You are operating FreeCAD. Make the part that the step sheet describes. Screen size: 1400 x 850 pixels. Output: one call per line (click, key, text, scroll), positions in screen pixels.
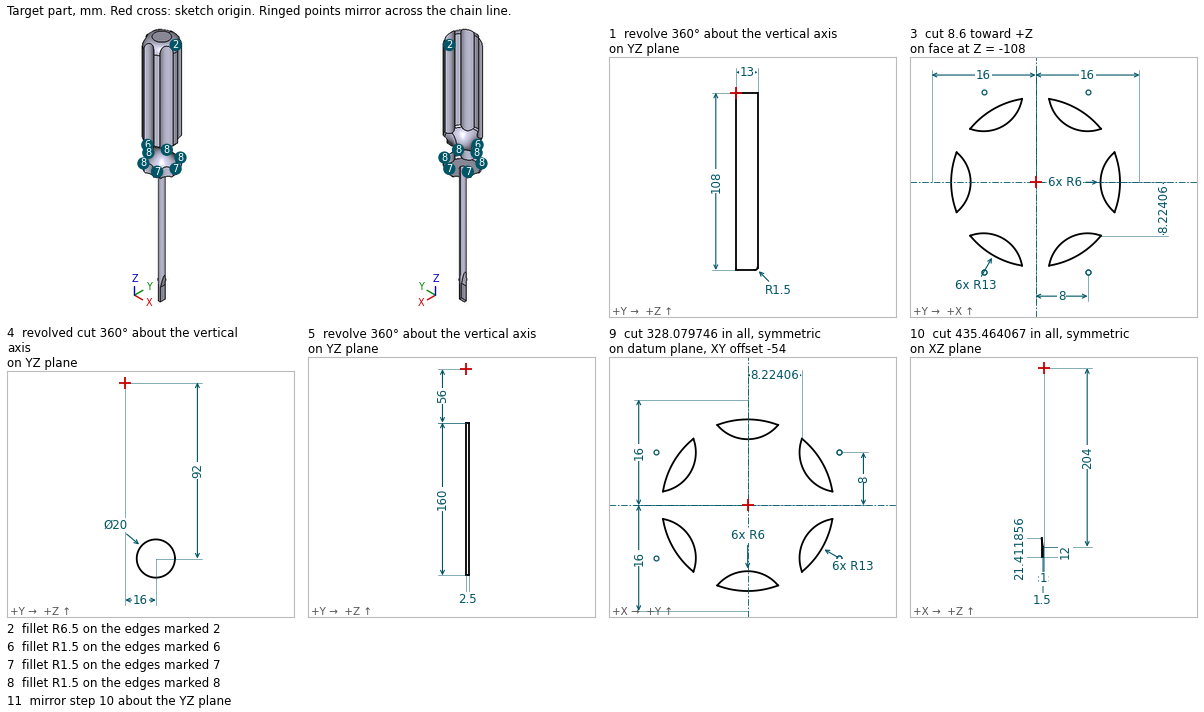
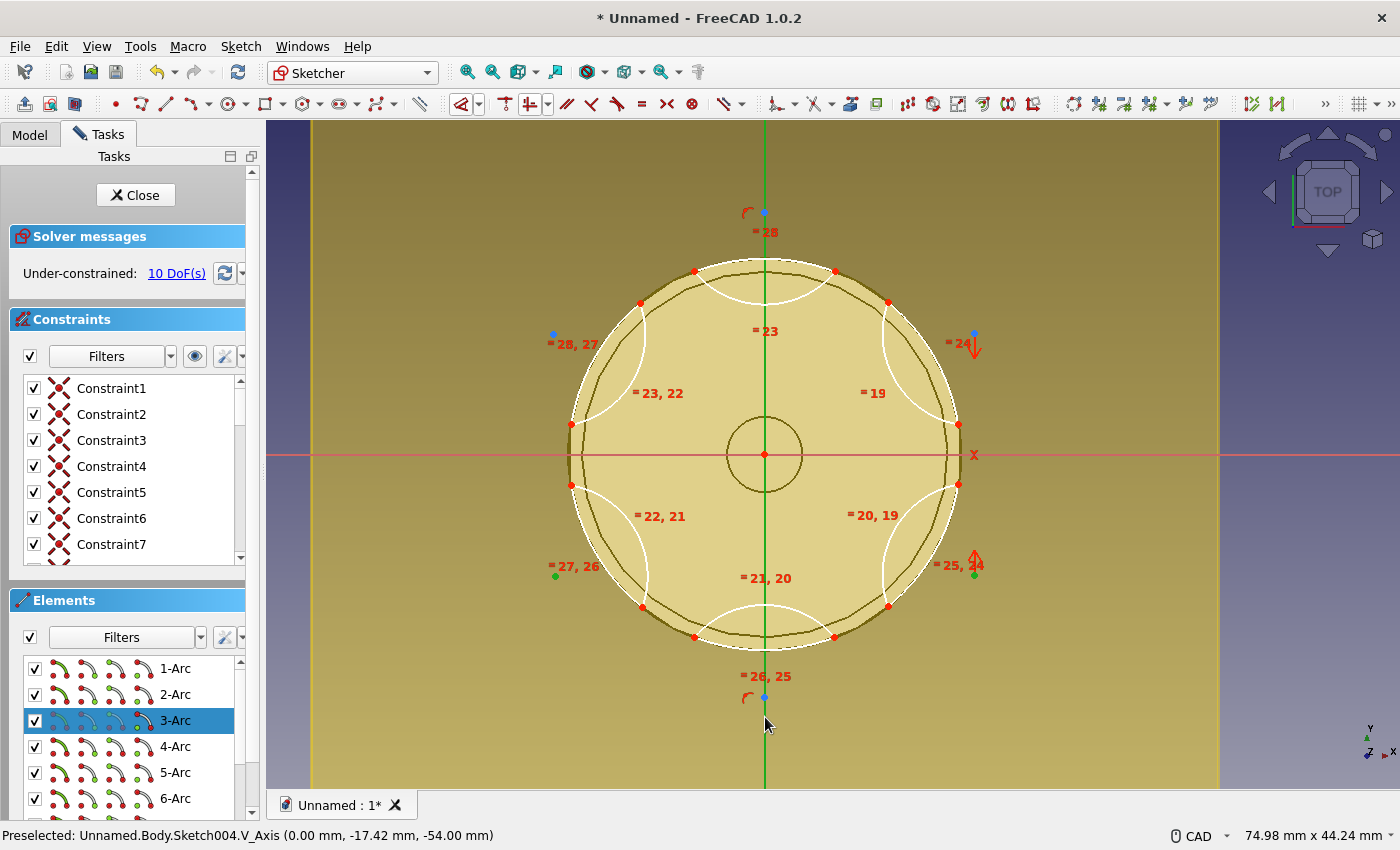
key(s)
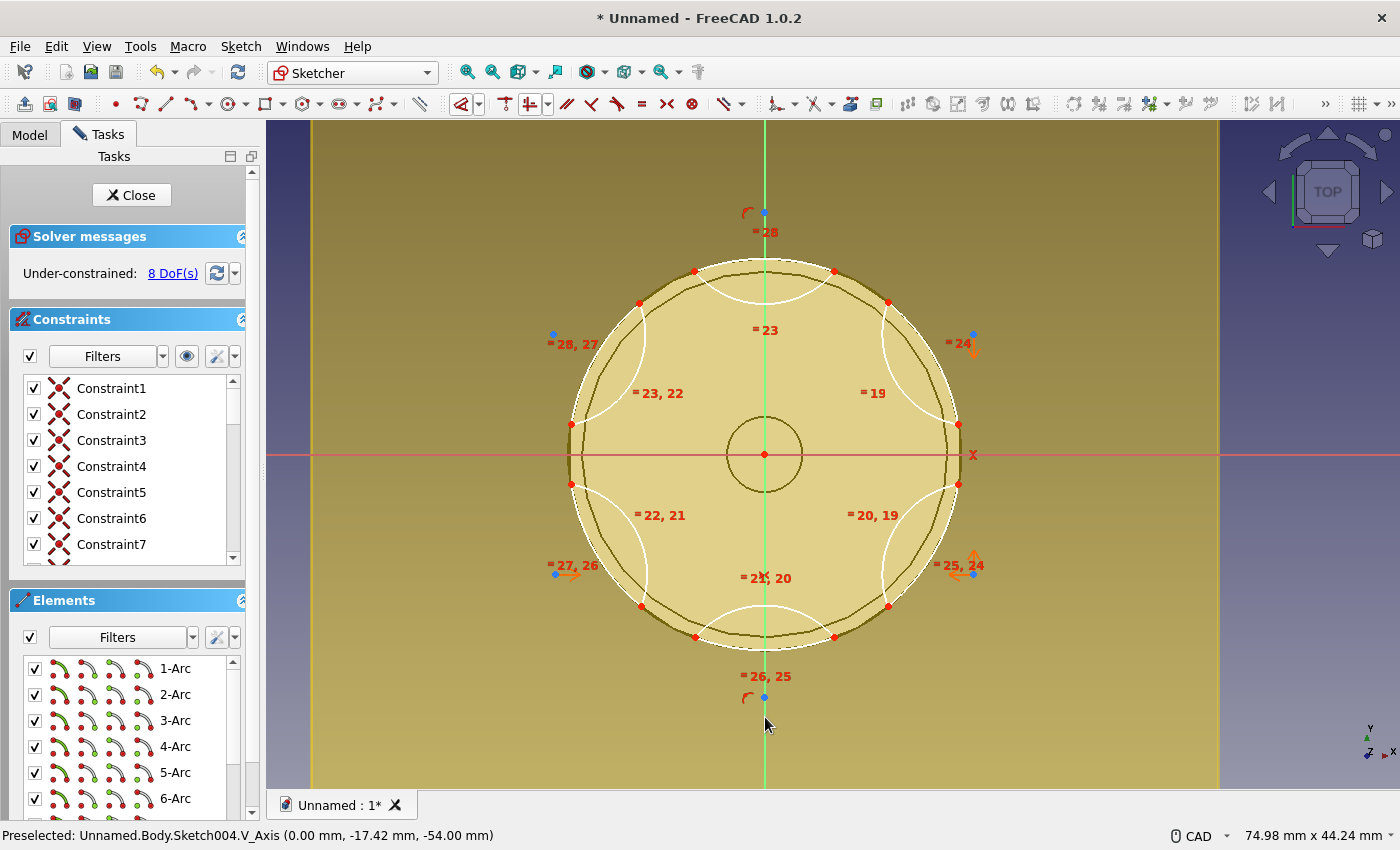
click(974, 334)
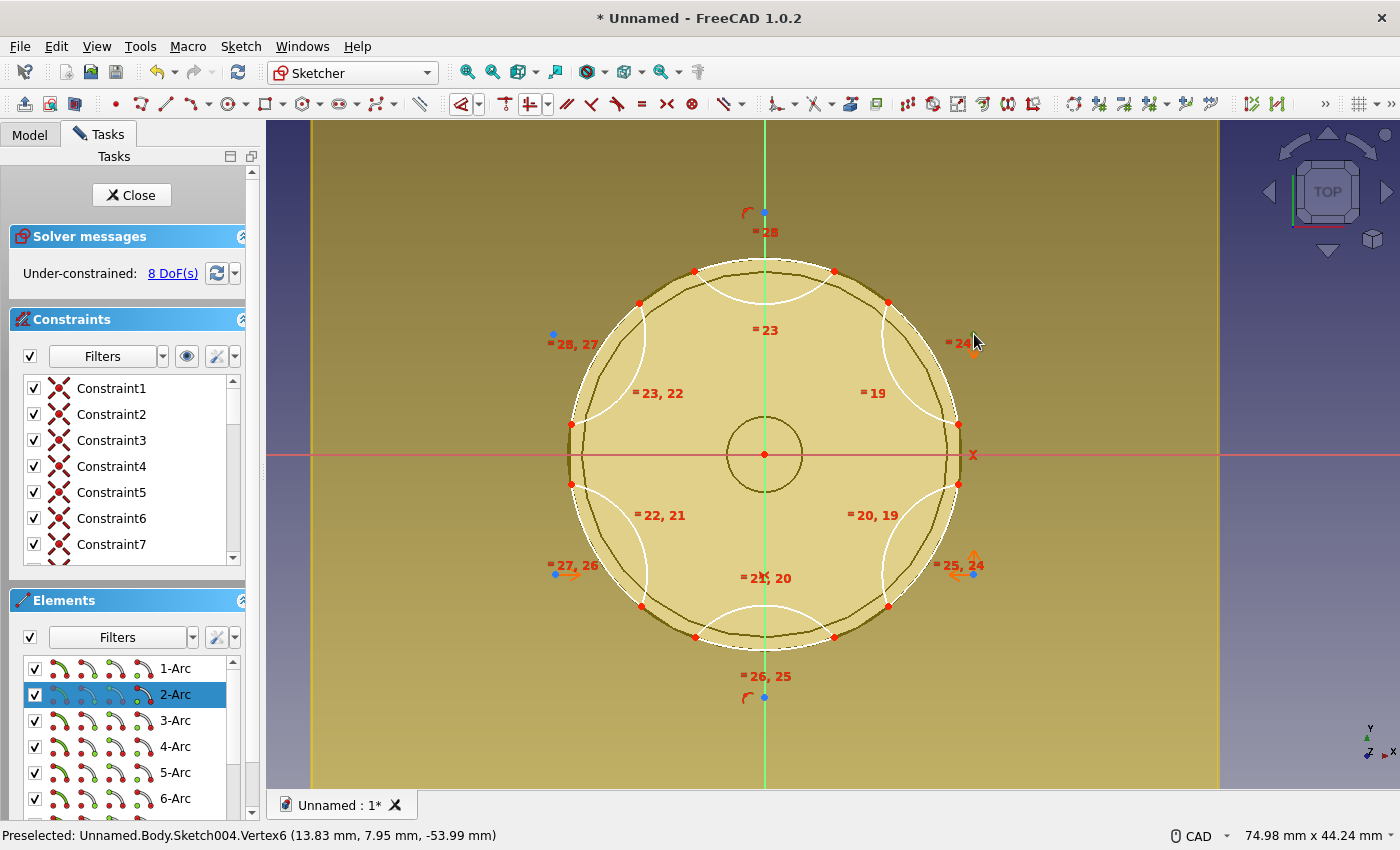
click(554, 335)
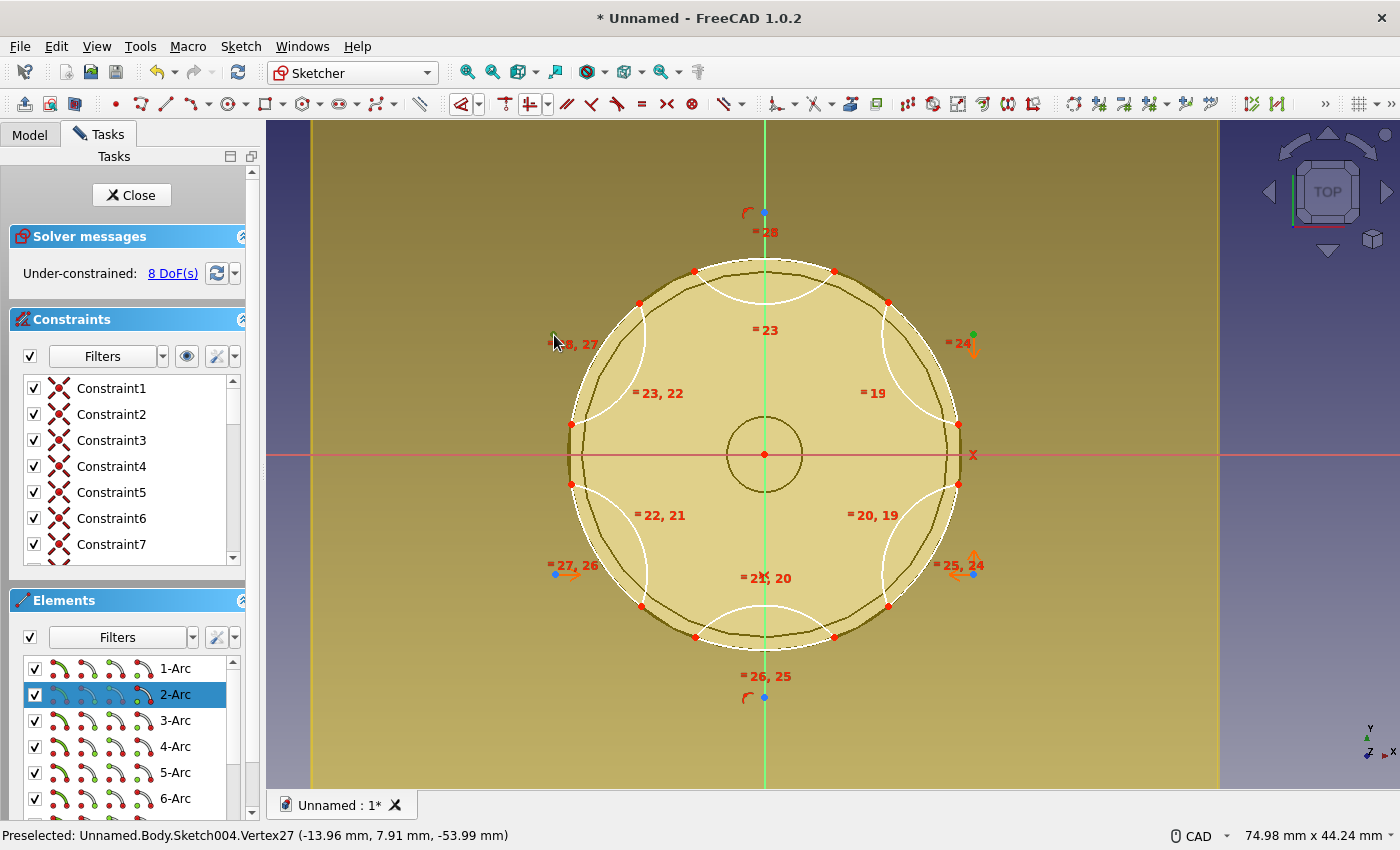
click(765, 717)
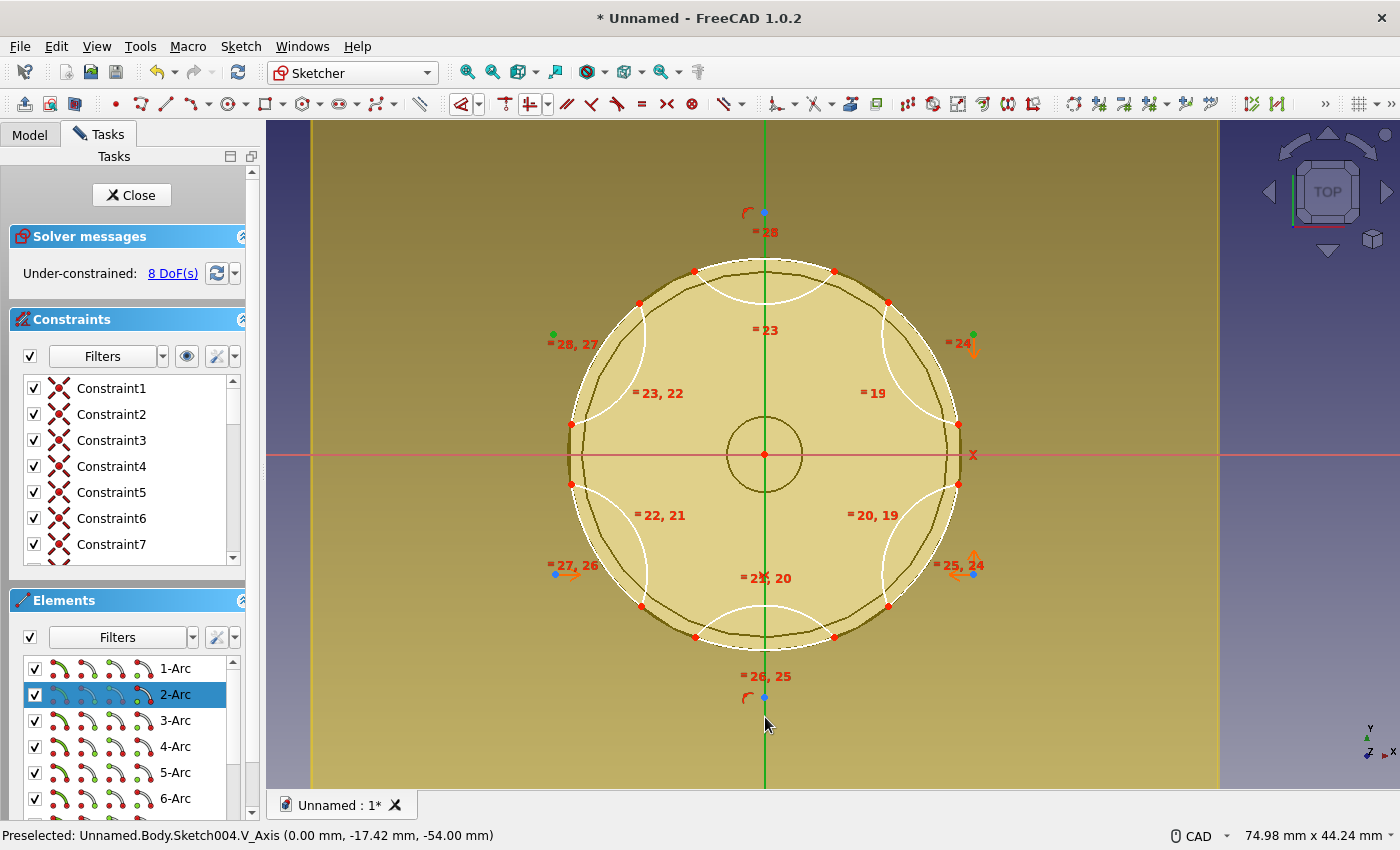
click(667, 104)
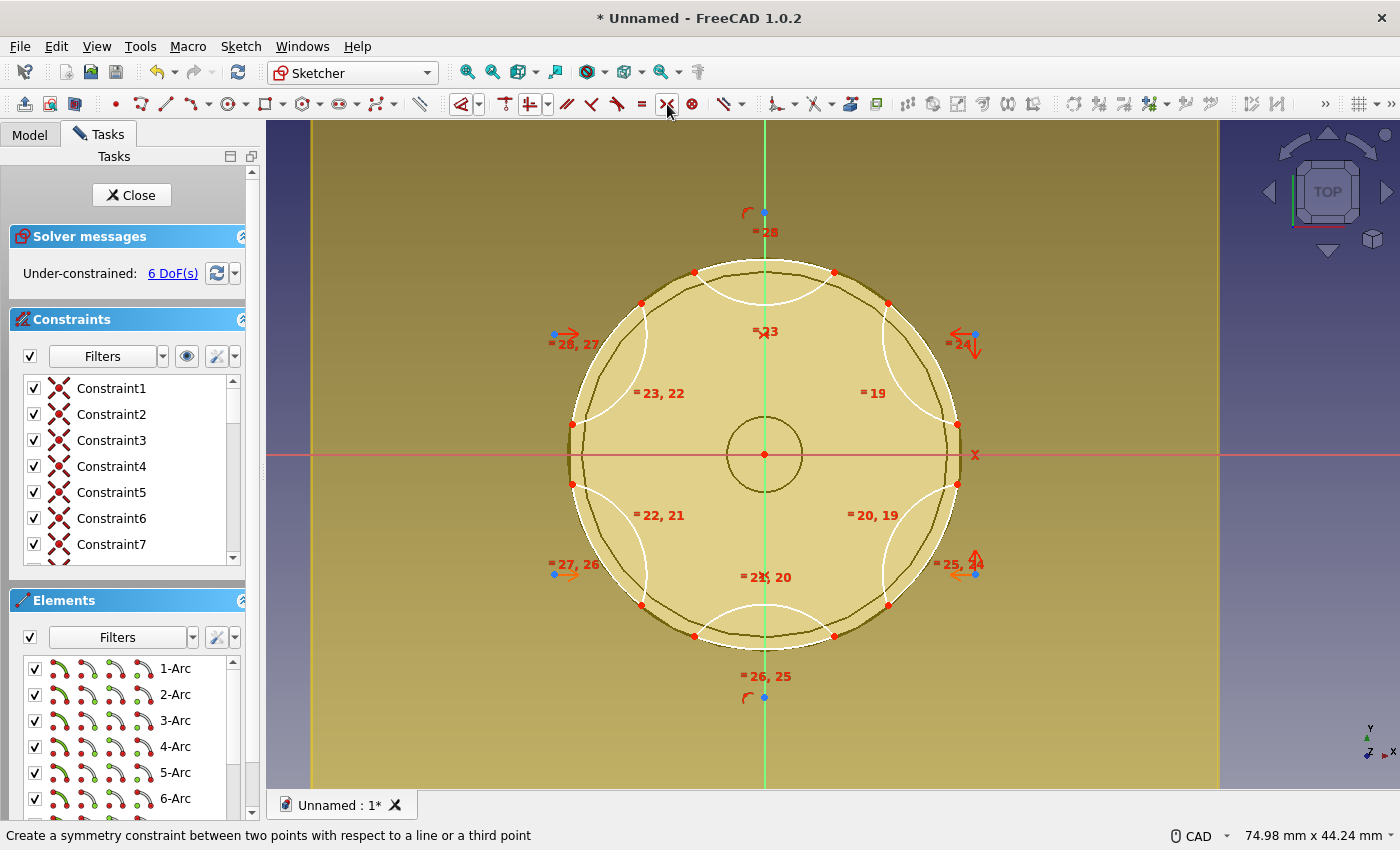
key(d)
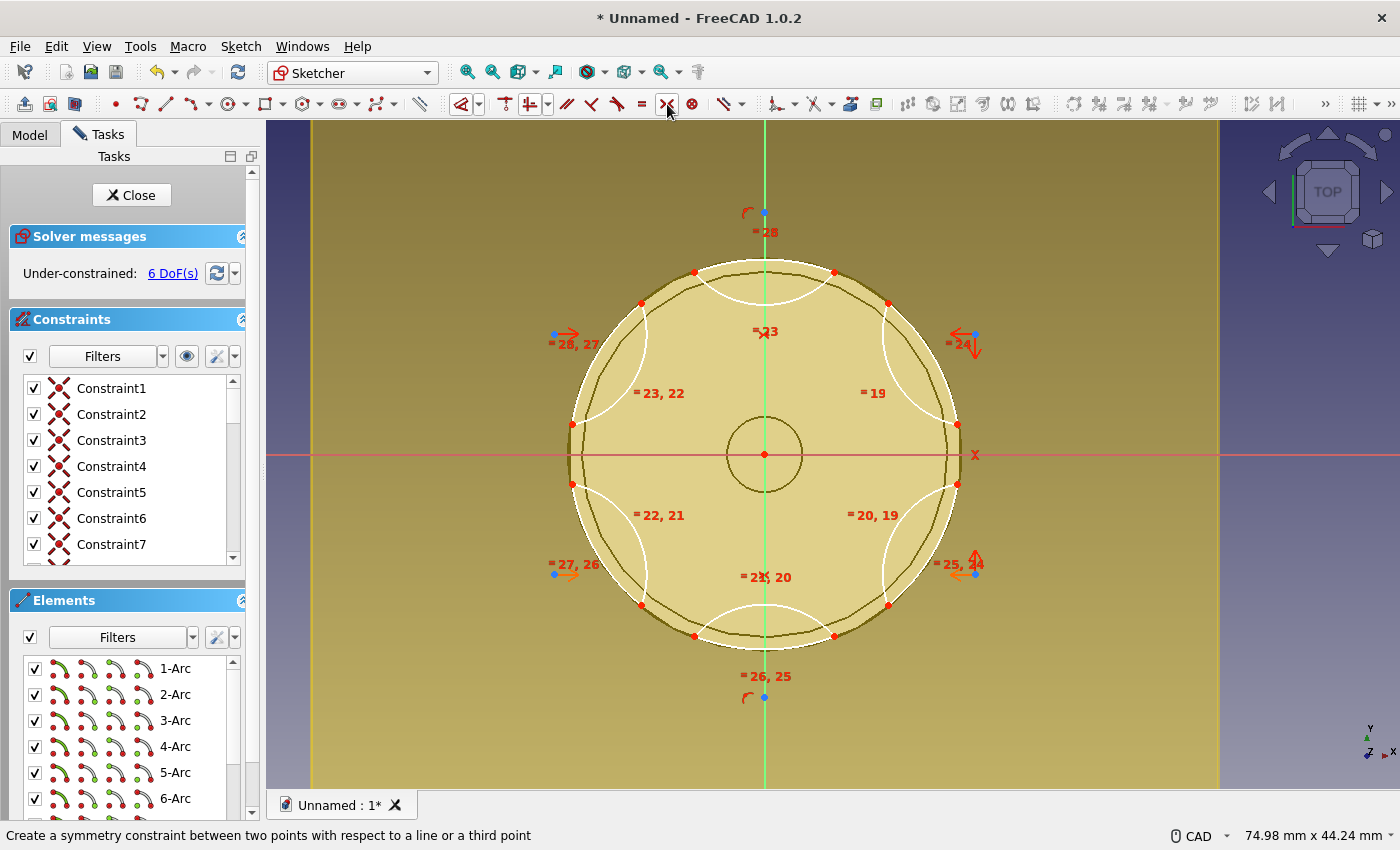
click(946, 383)
click(976, 371)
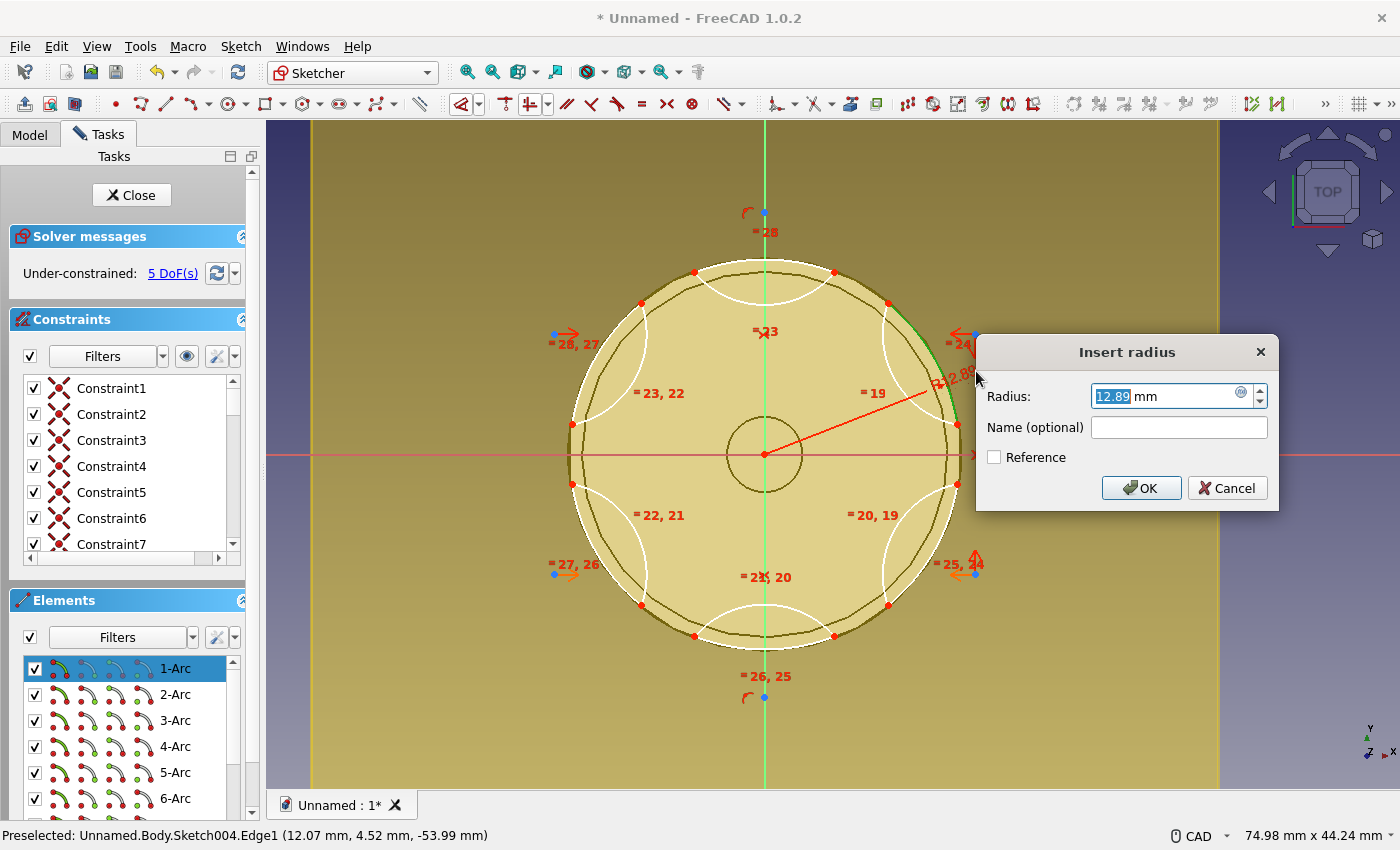
text(13)
key(Return)